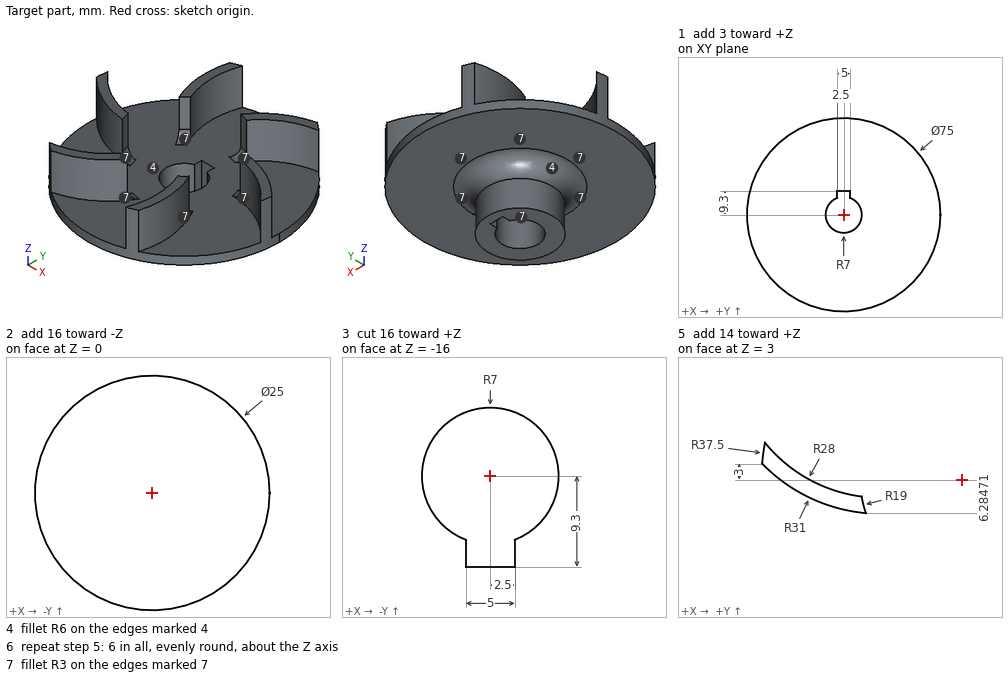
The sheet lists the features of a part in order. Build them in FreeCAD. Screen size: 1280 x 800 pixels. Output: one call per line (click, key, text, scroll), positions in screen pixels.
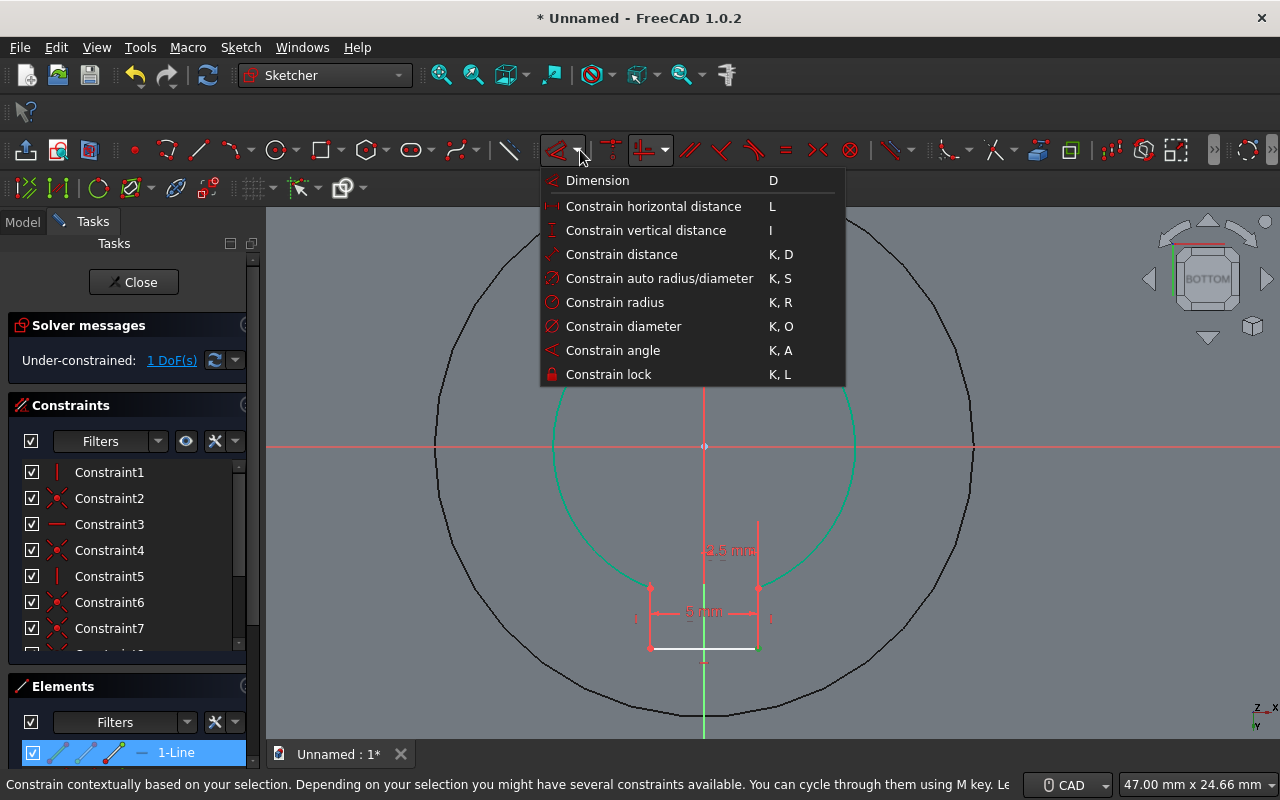
click(693, 230)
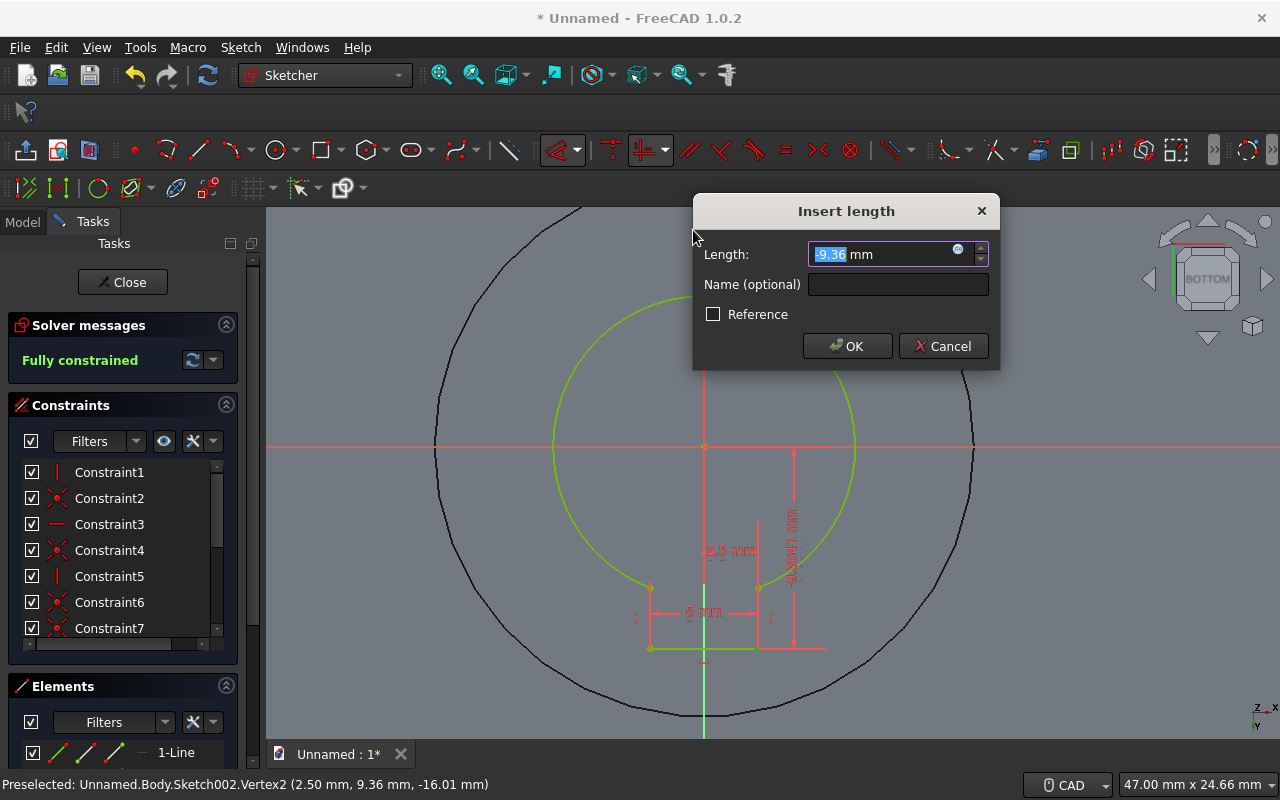
text(-9.3)
key(Return)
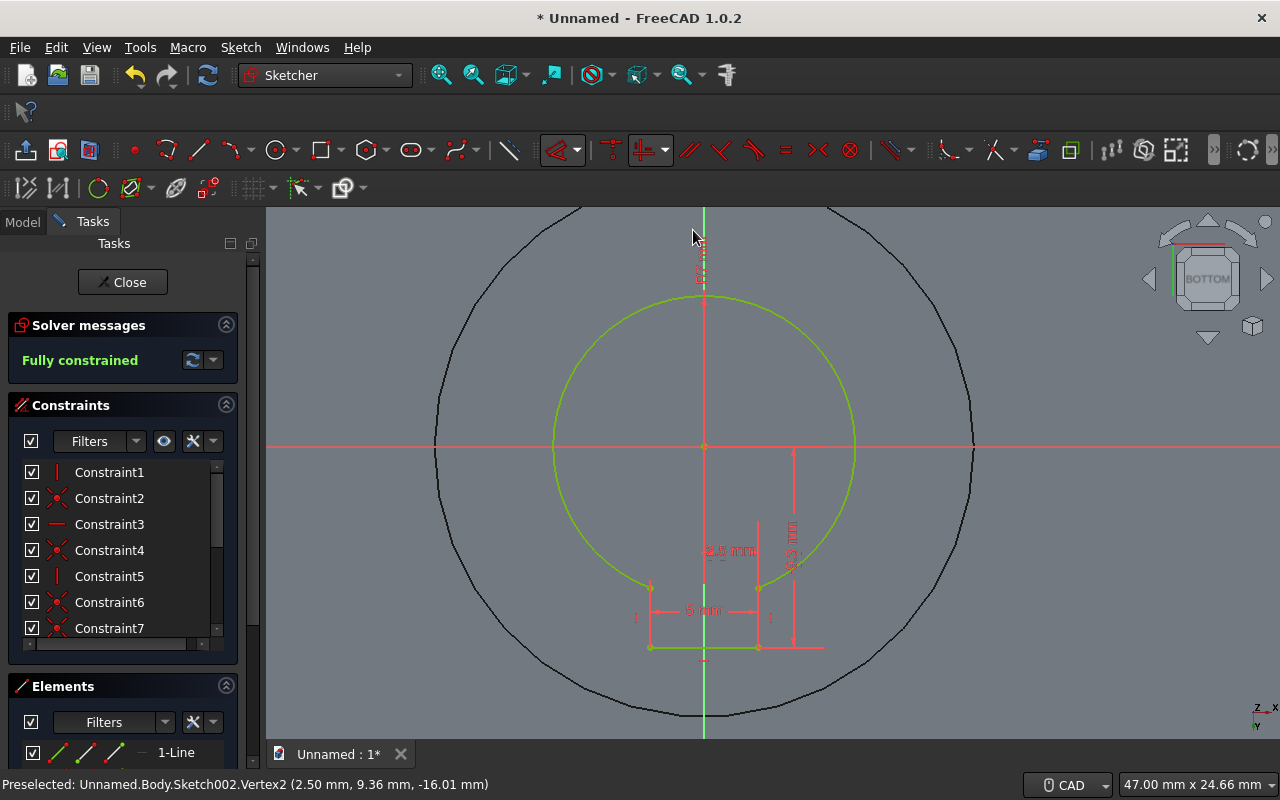
click(123, 282)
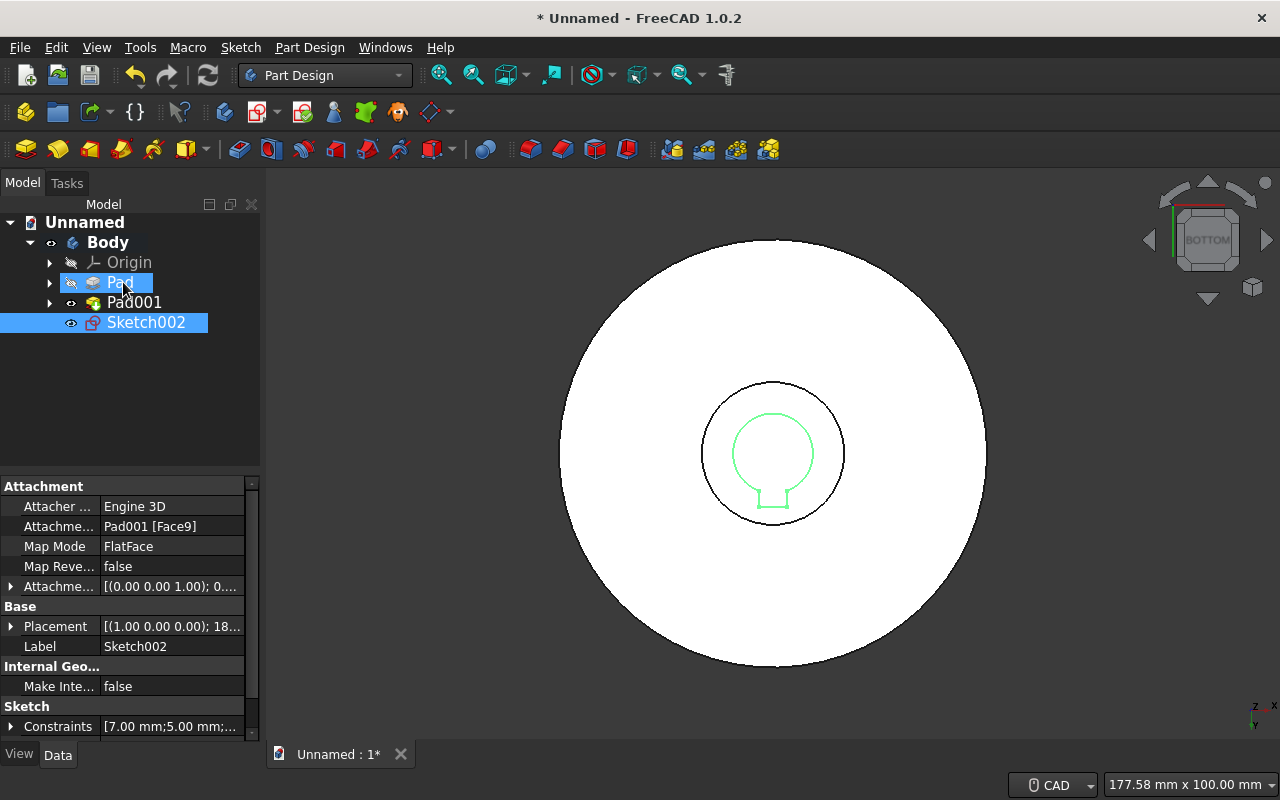
click(240, 150)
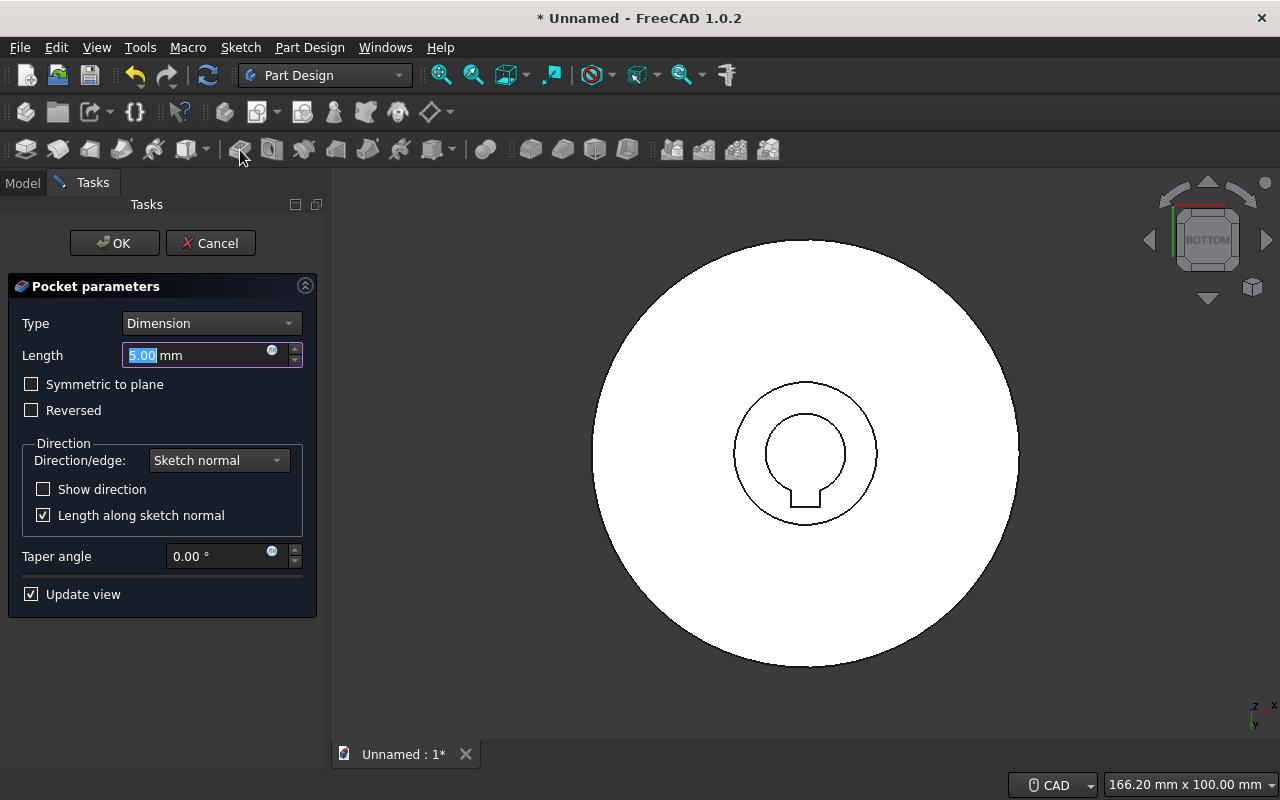
text(16)
key(Tab)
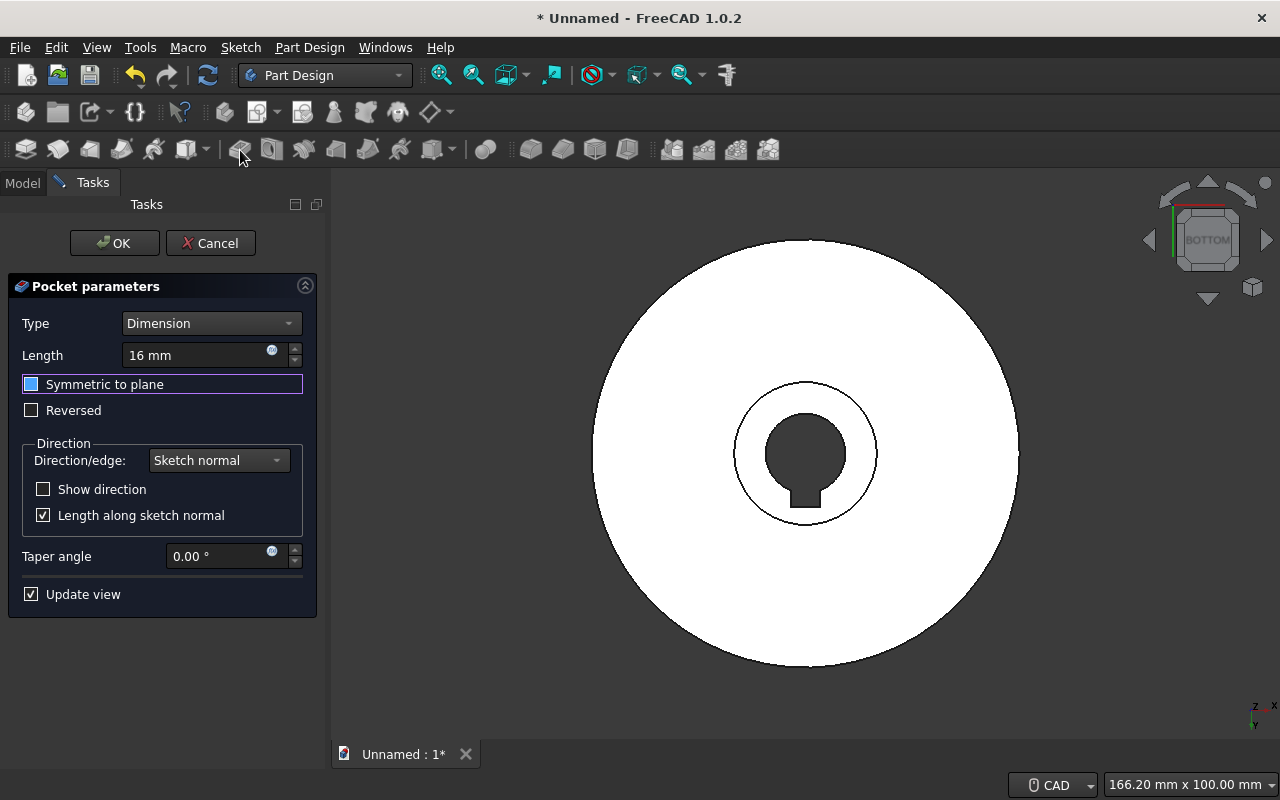
click(115, 243)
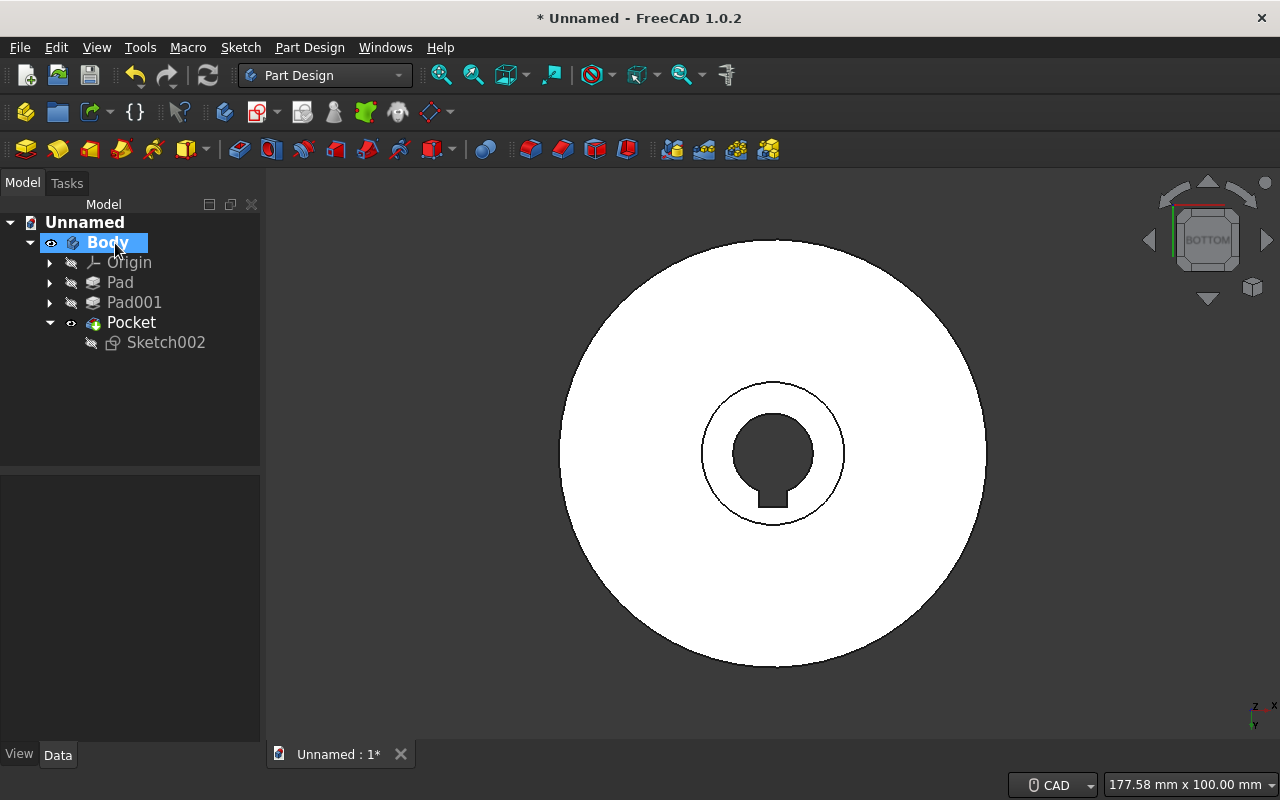
key(0)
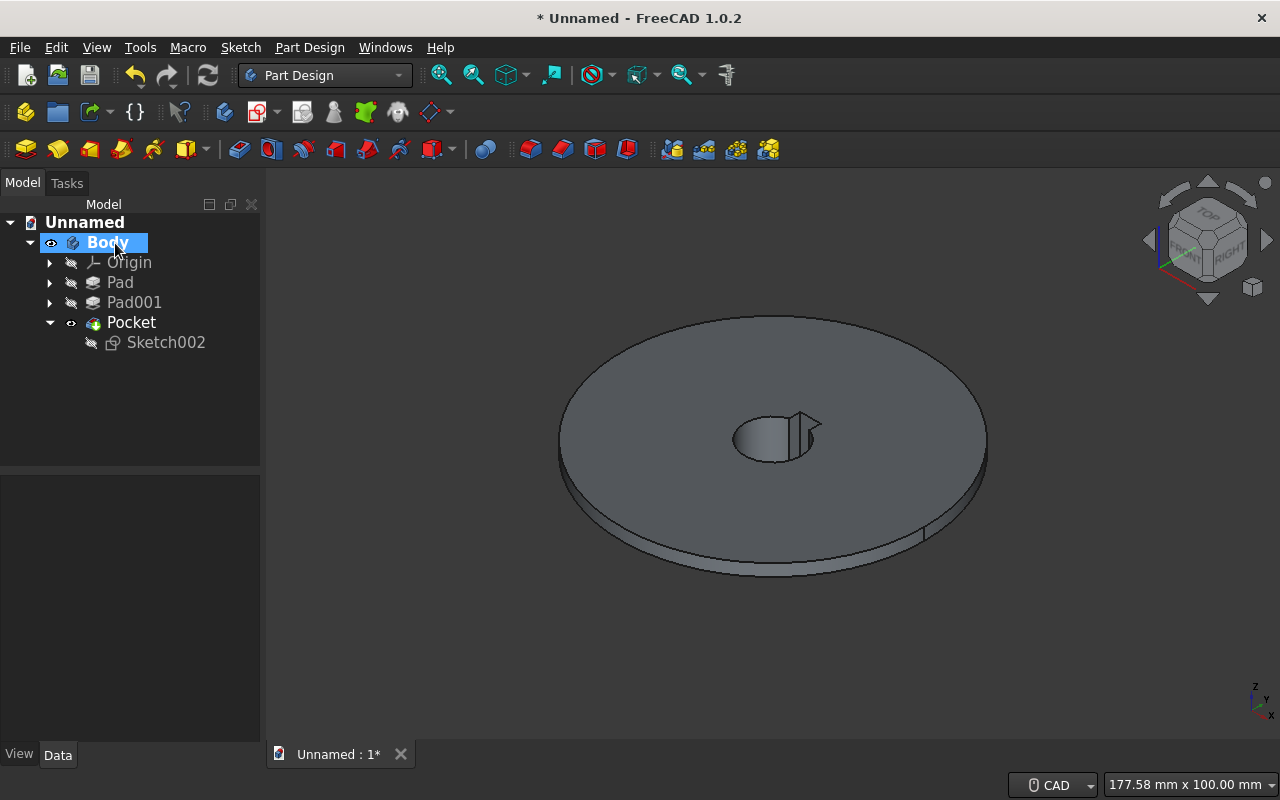
key(2)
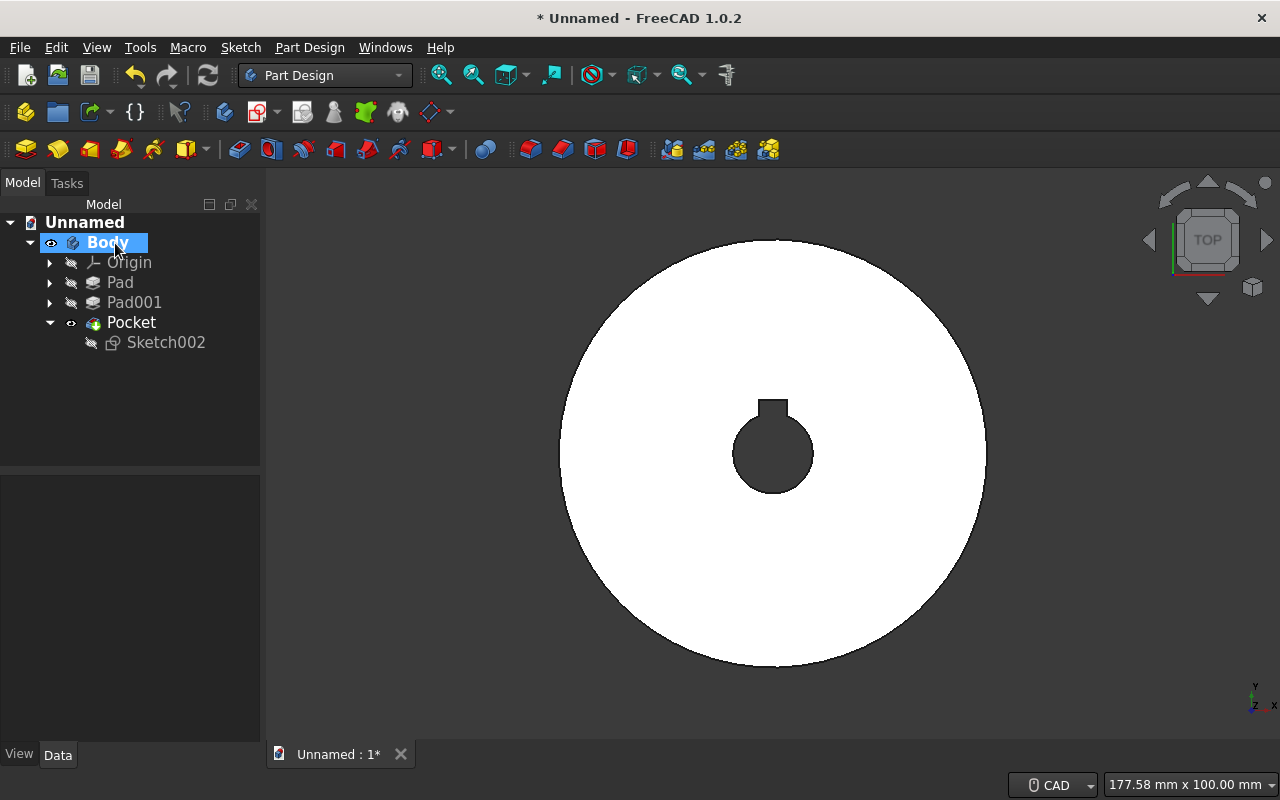
key(1)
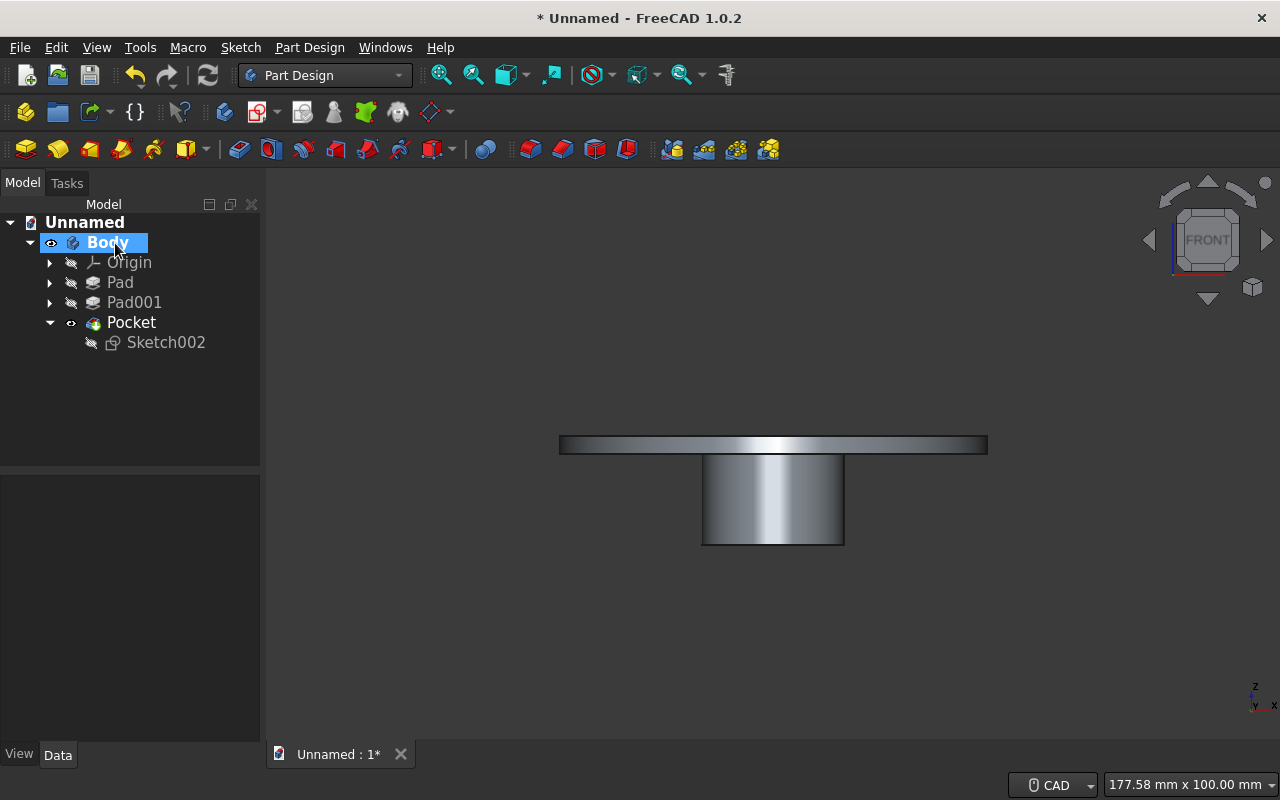
key(v)
key(f)